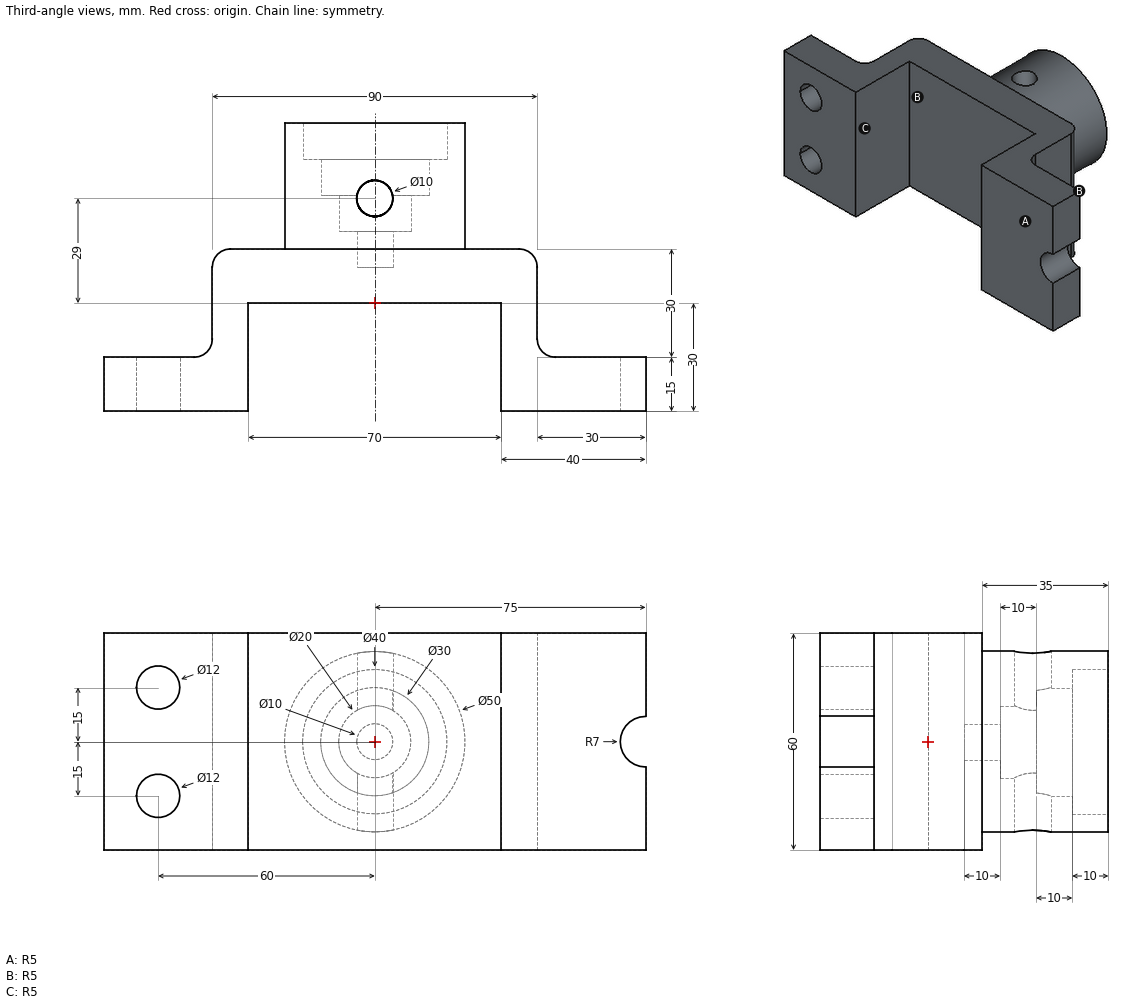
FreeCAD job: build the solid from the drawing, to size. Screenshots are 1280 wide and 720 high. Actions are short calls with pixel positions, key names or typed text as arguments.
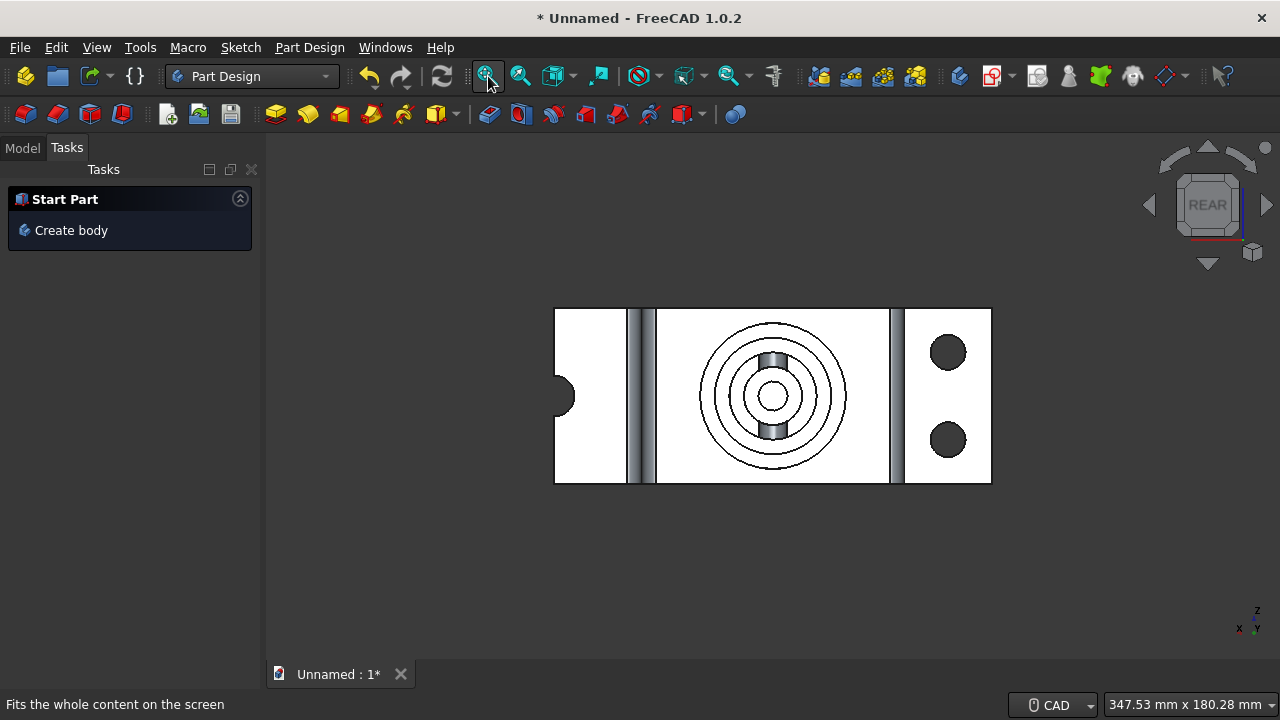
key(6)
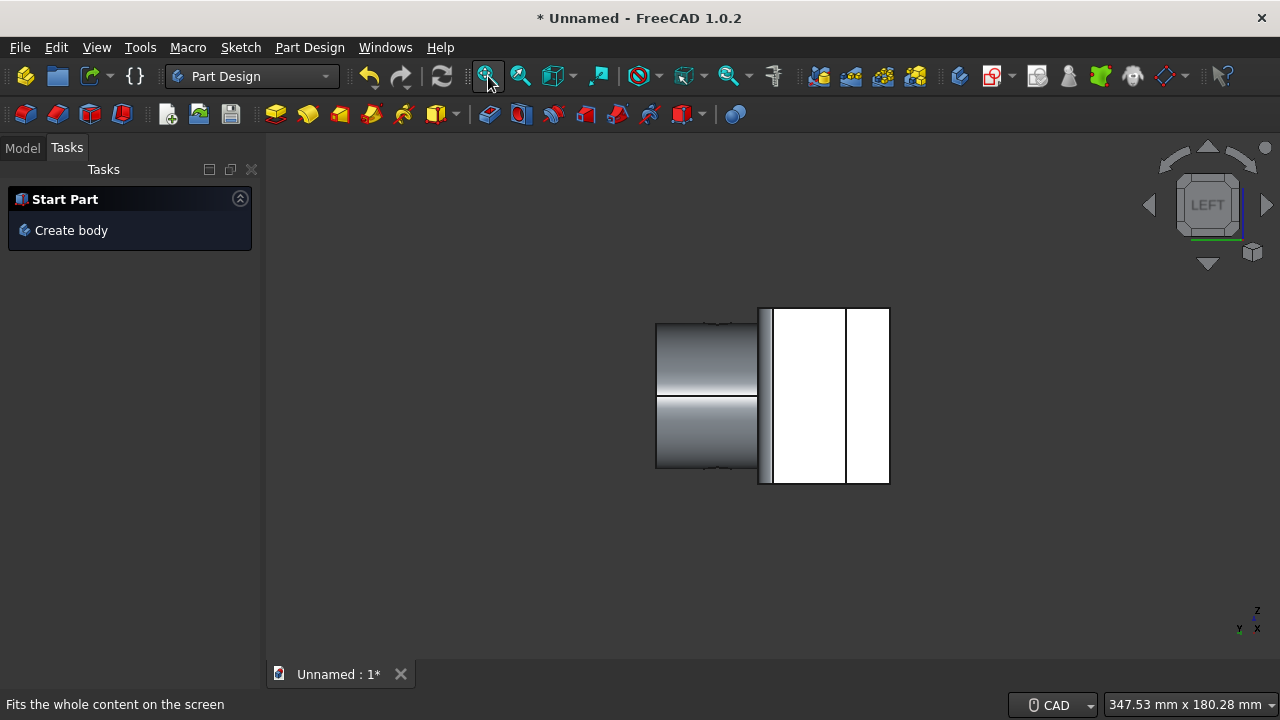
click(488, 76)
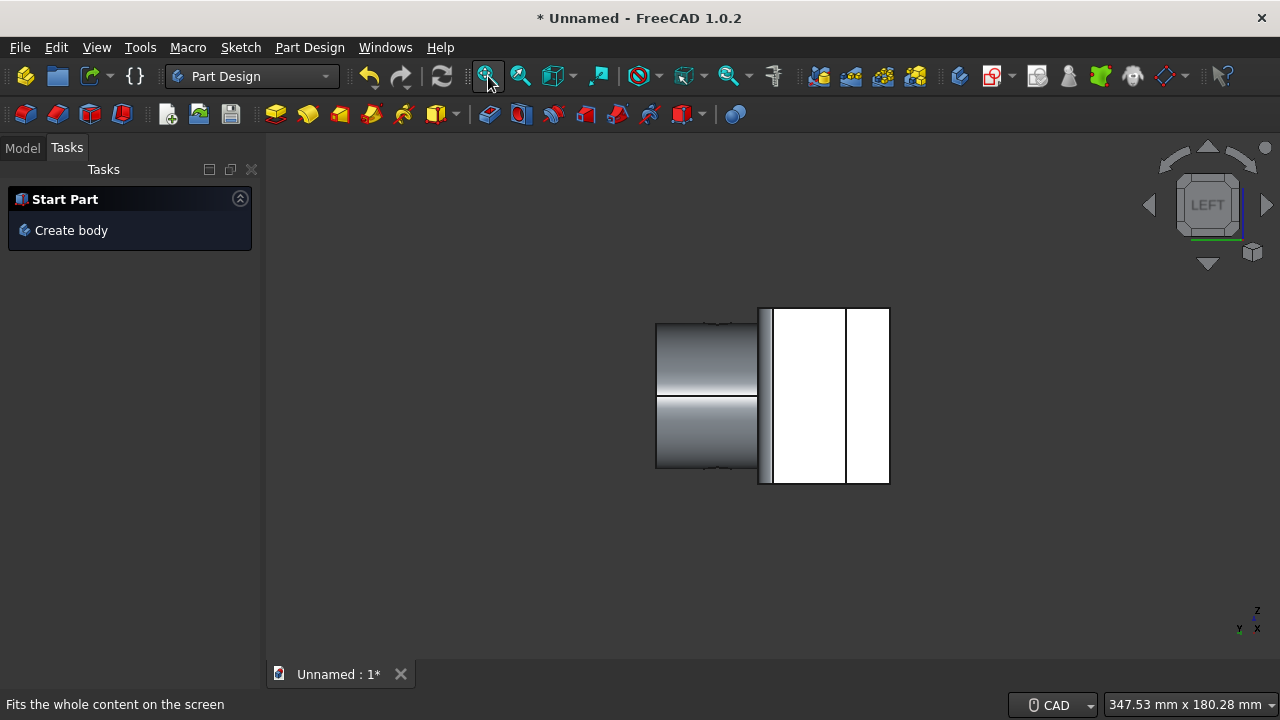
key(v)
key(3)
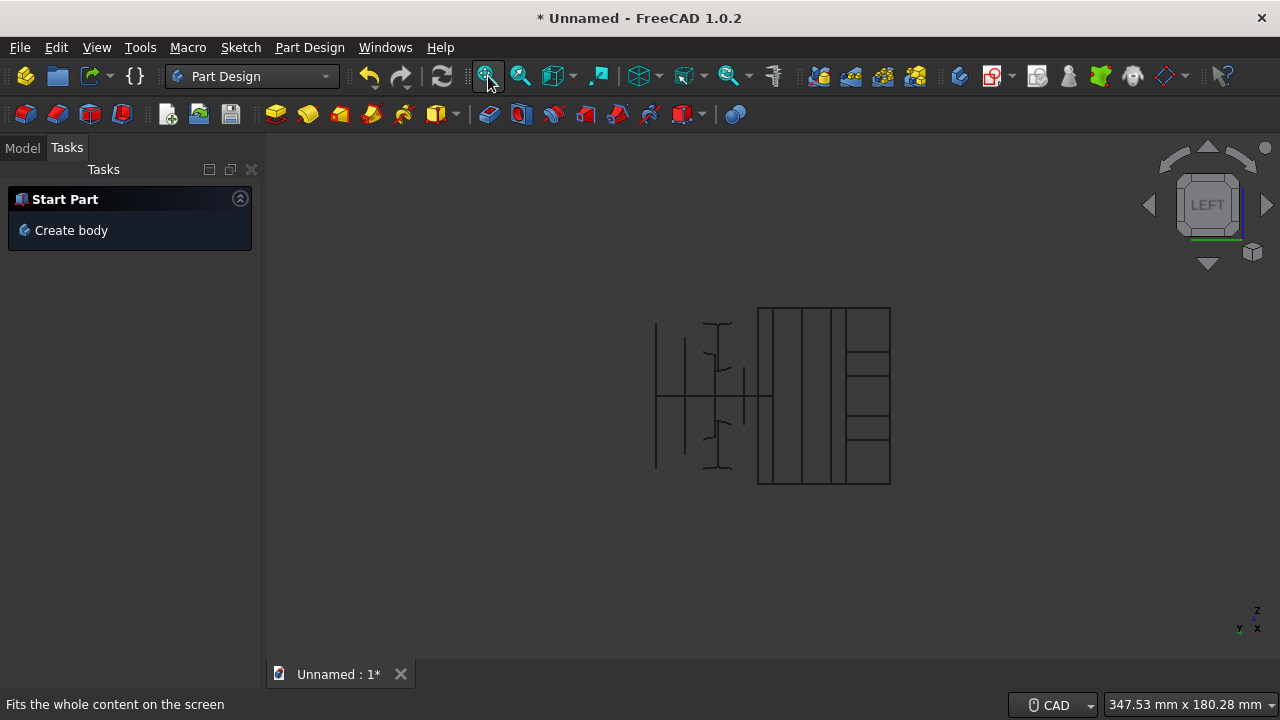
key(0)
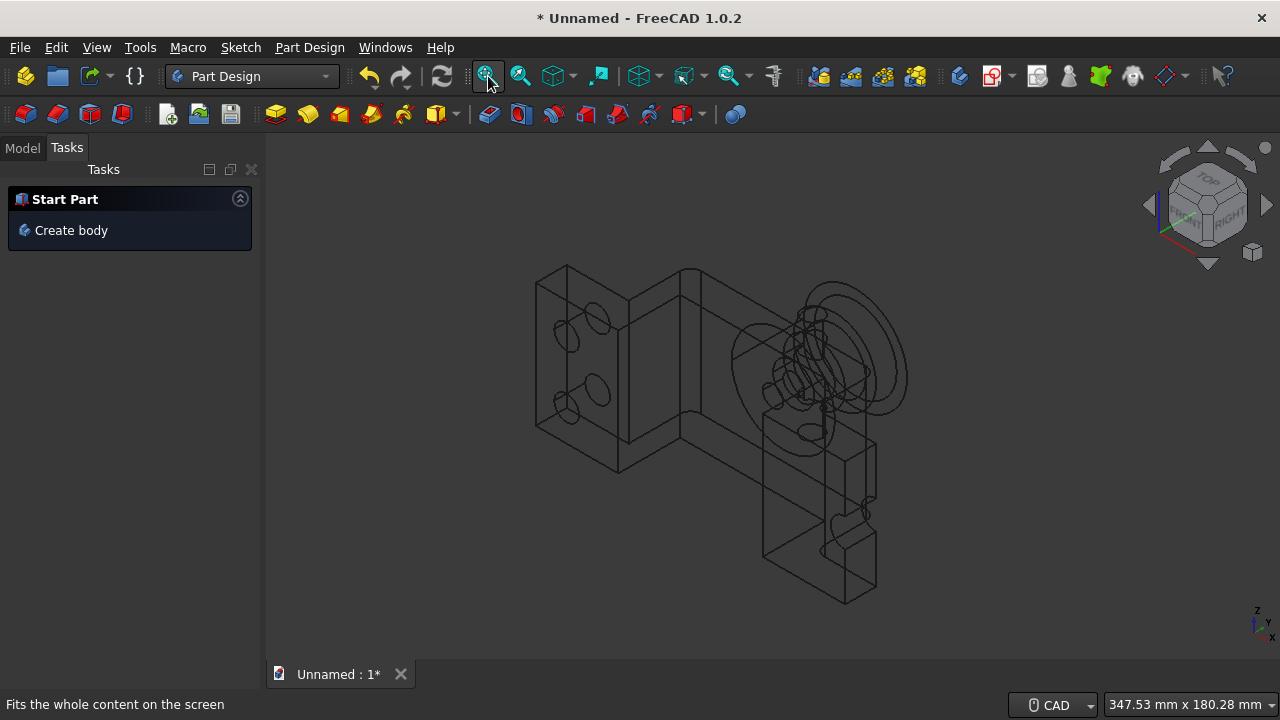
click(629, 371)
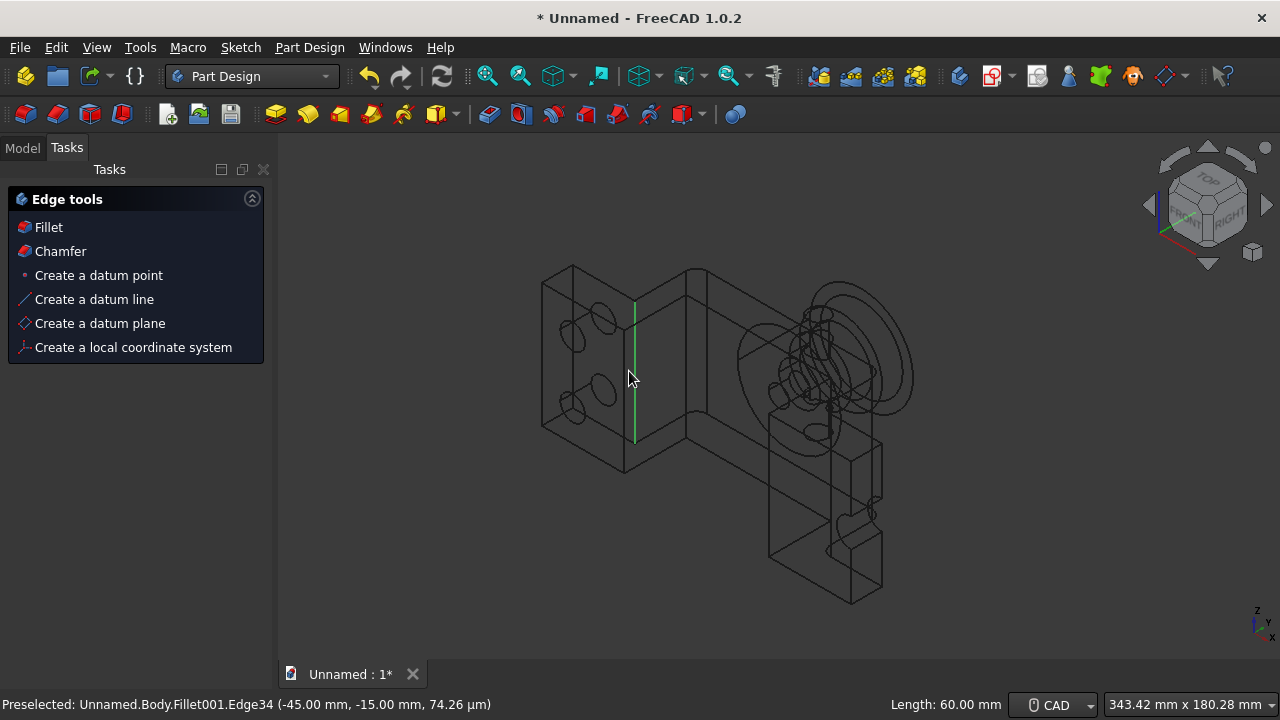
key(v)
key(1)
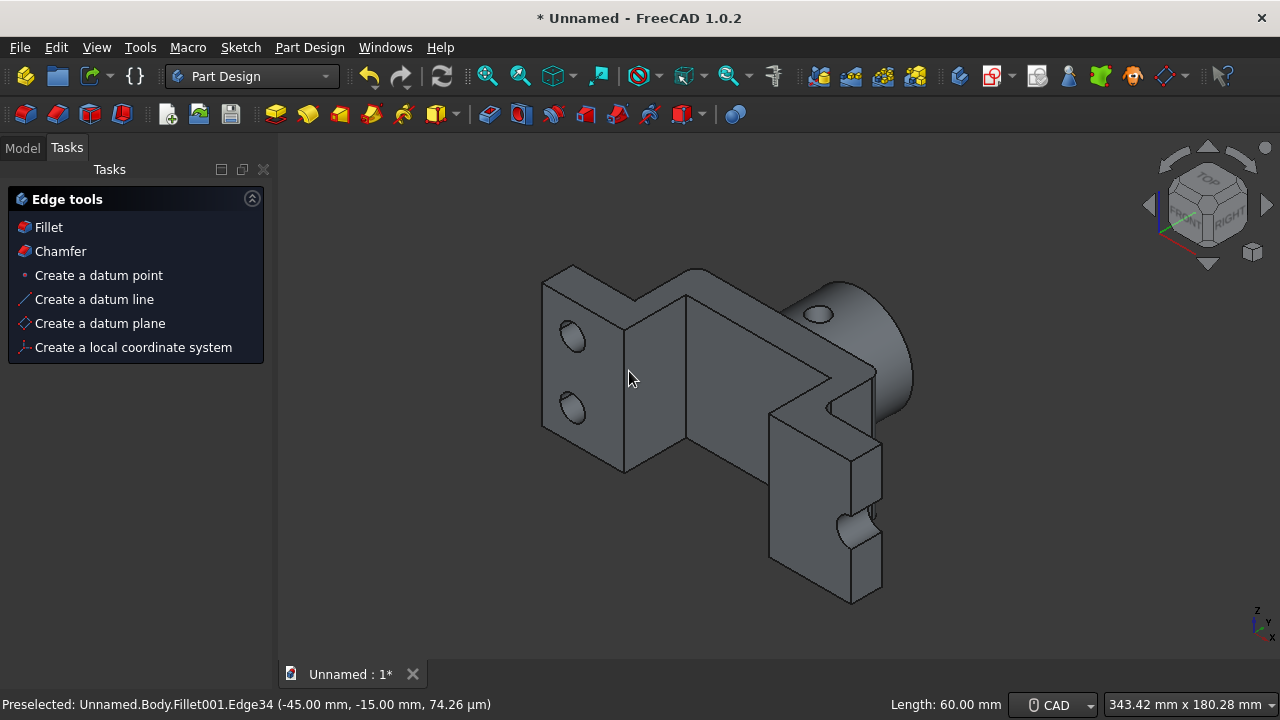
click(26, 114)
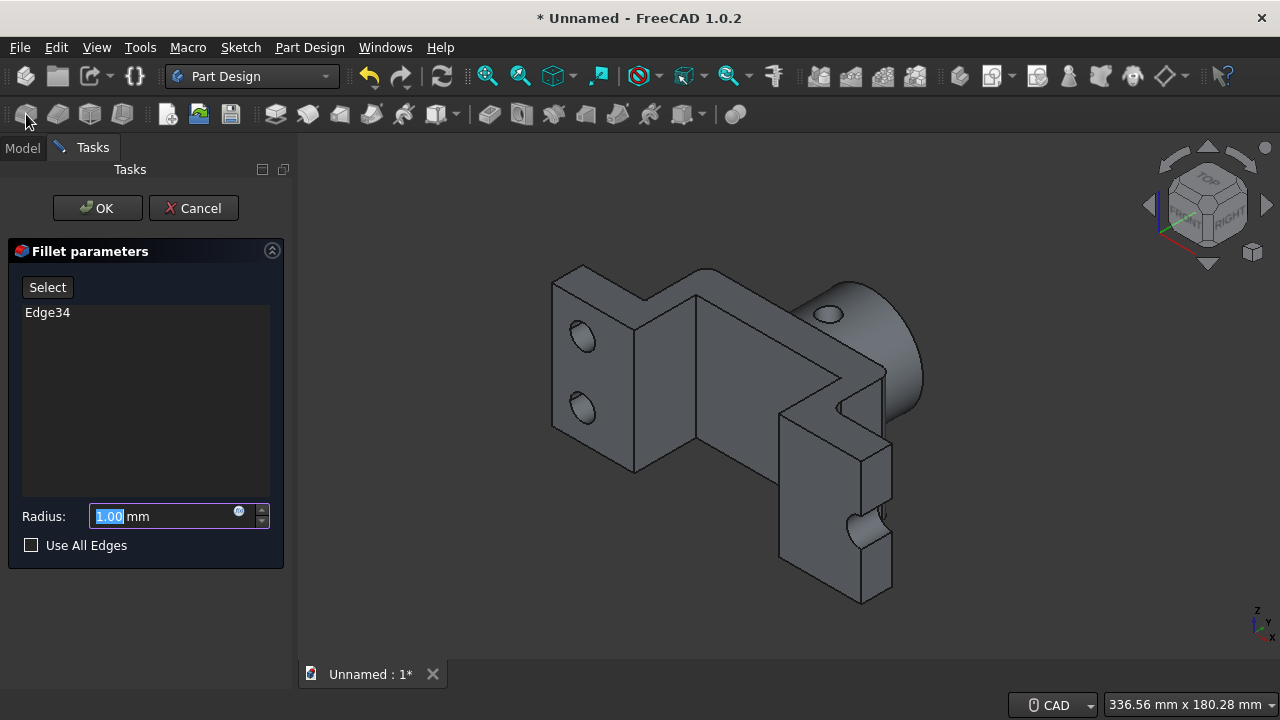
text(5)
key(Tab)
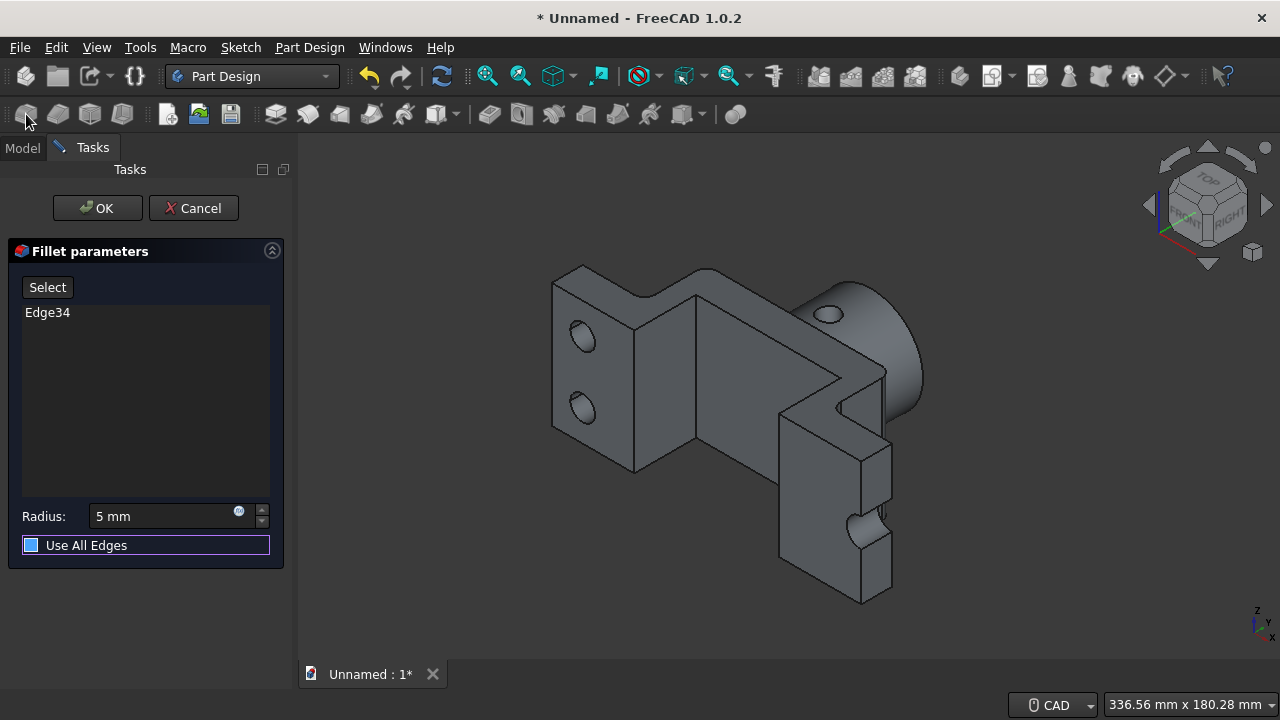
click(98, 208)